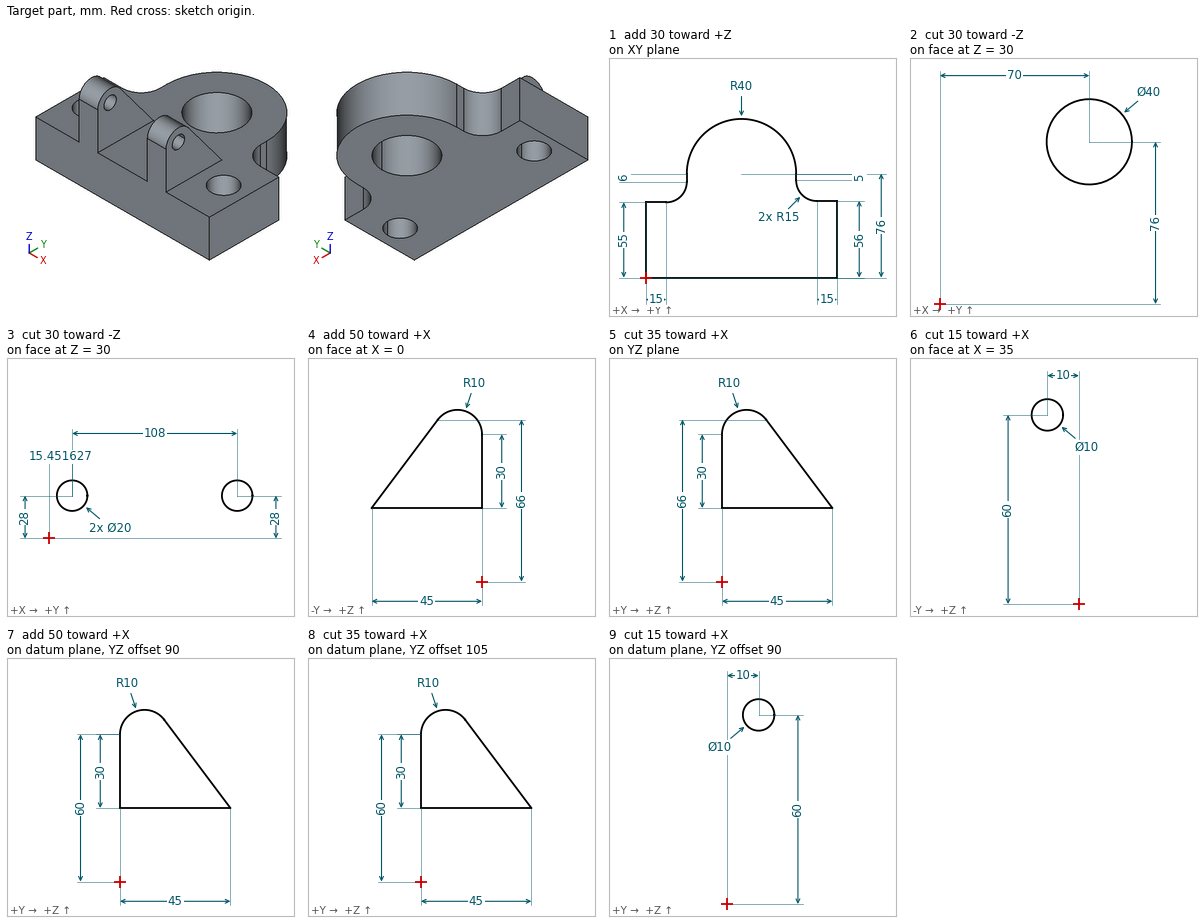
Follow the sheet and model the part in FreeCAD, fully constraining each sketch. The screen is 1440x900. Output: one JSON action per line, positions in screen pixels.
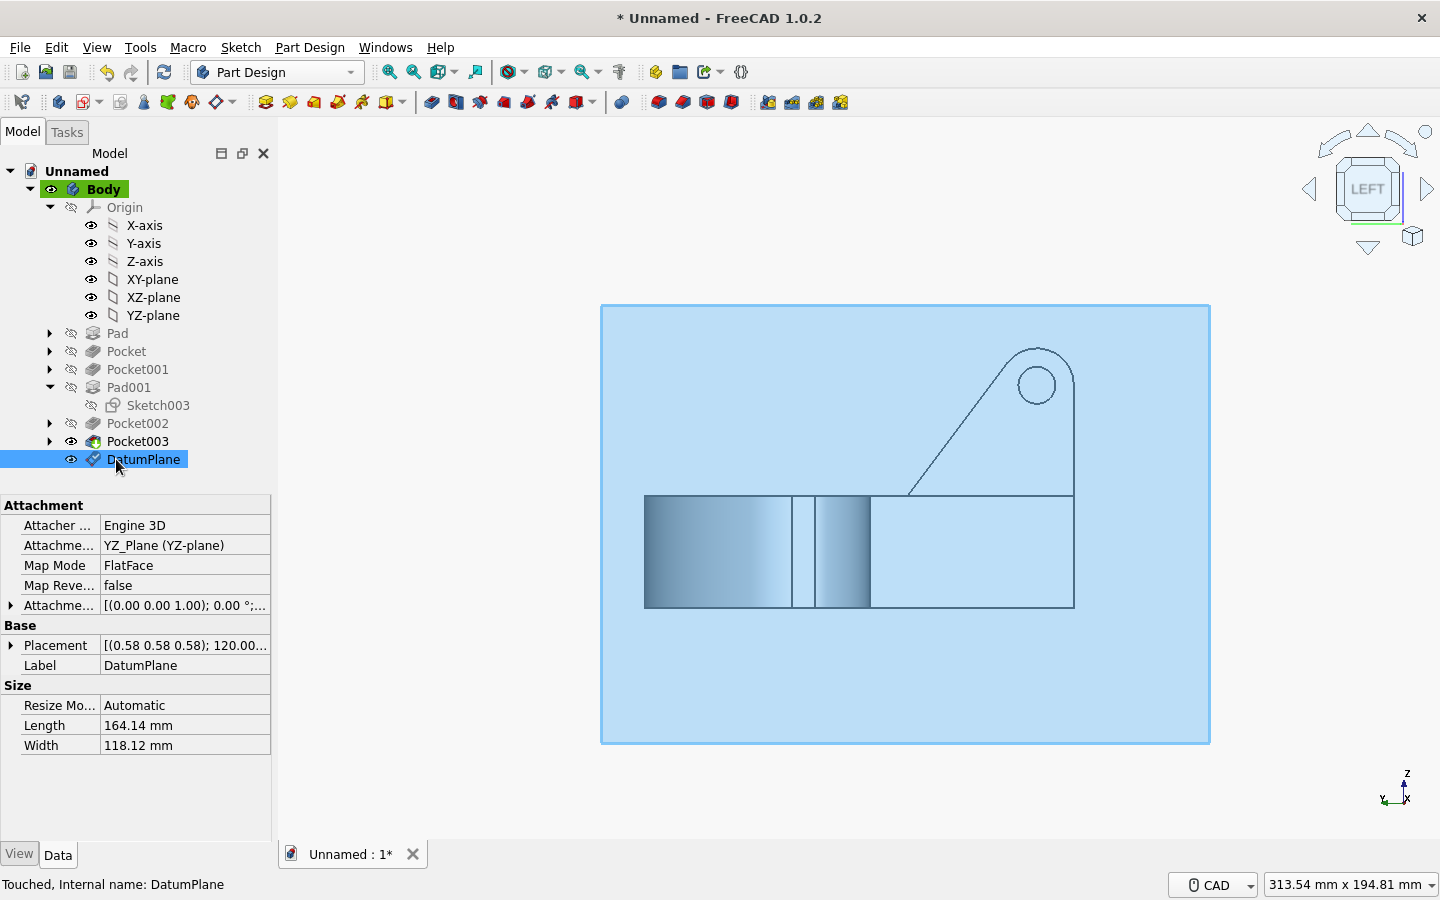
{"action": "left_click", "coordinate": [84, 102]}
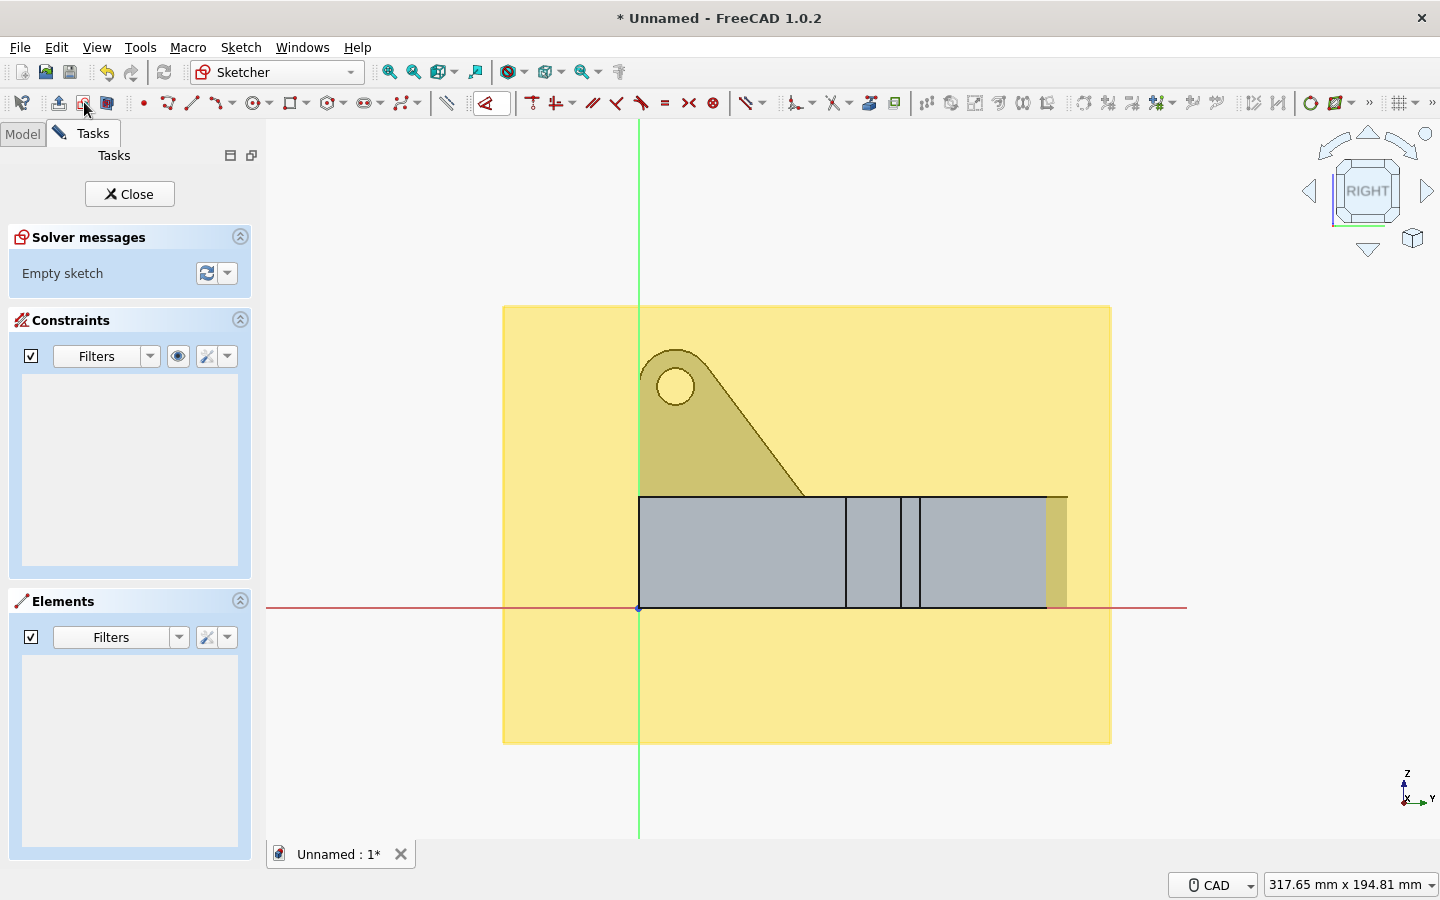
{"action": "left_click", "coordinate": [108, 104]}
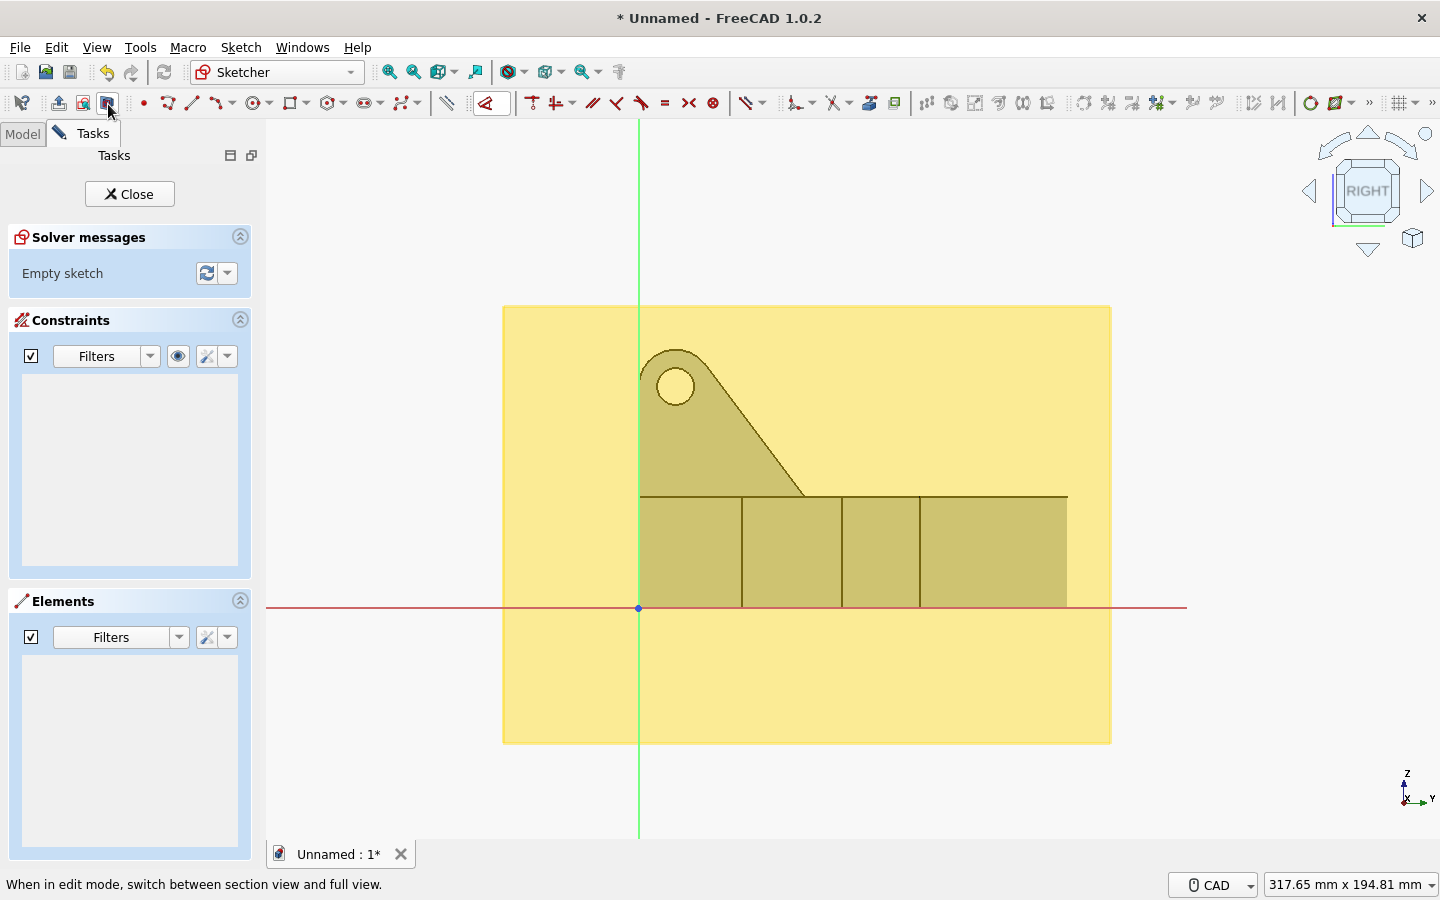
{"action": "scroll", "coordinate": [646, 481], "scroll_direction": "up", "scroll_amount": 3}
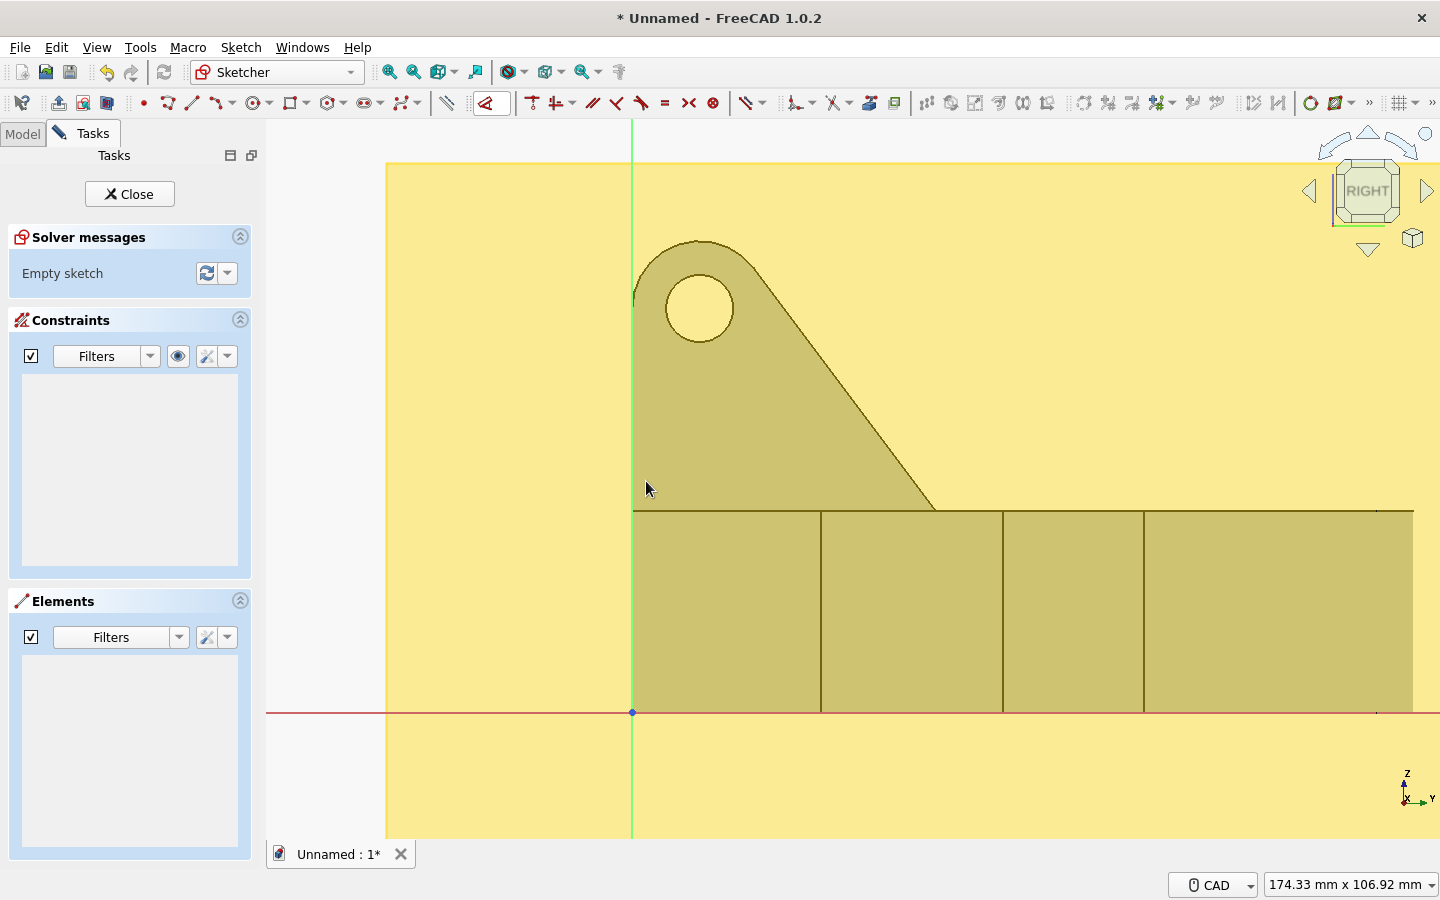
{"action": "key", "text": "g m"}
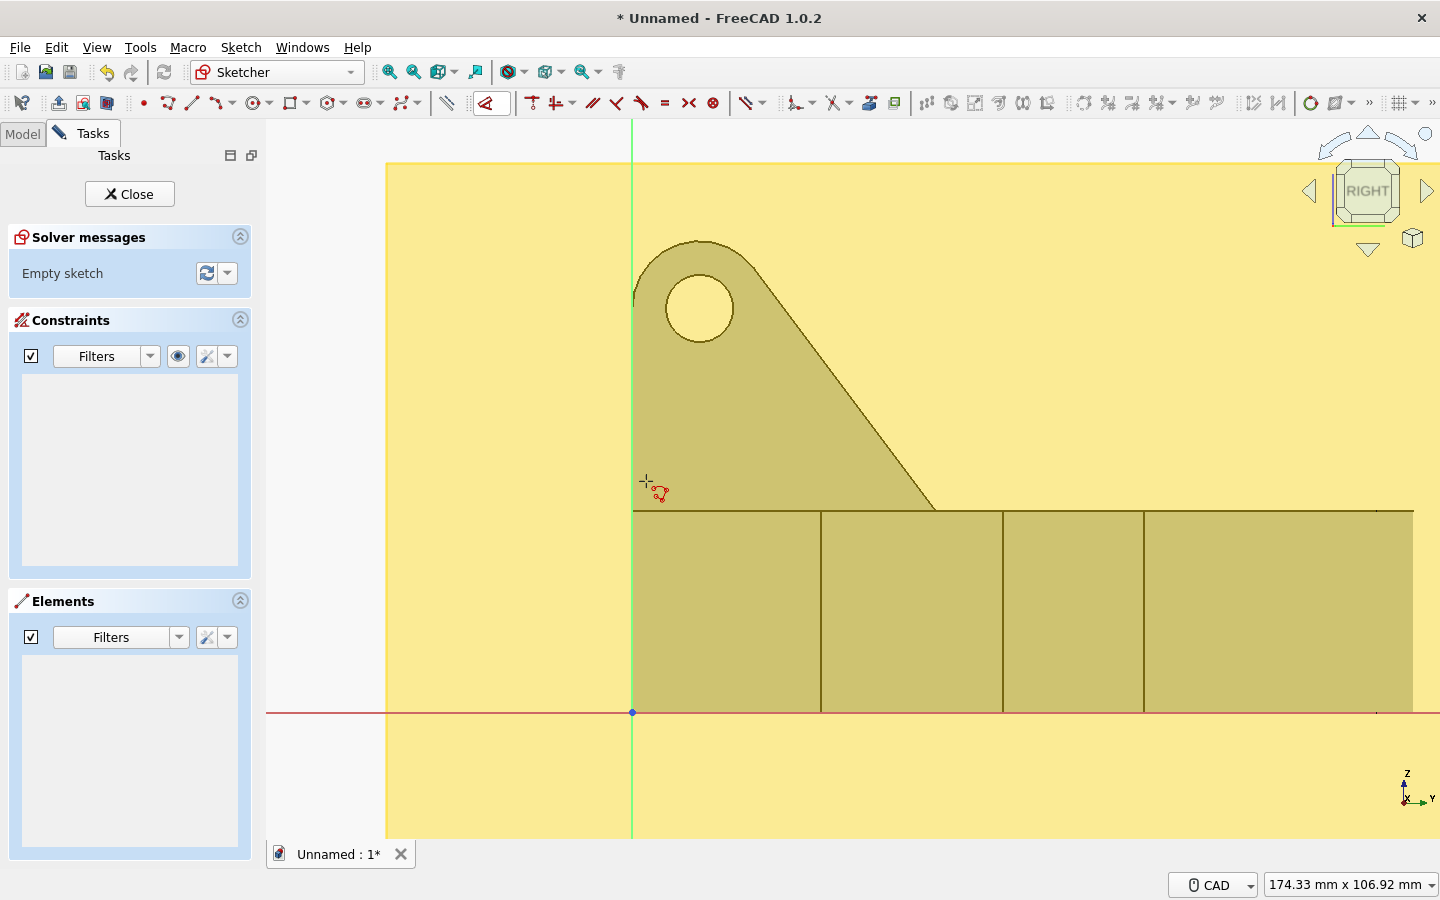
{"action": "left_click", "coordinate": [632, 308]}
{"action": "left_click", "coordinate": [641, 511]}
{"action": "left_click", "coordinate": [935, 511]}
{"action": "left_click", "coordinate": [754, 268]}
{"action": "right_click", "coordinate": [754, 268]}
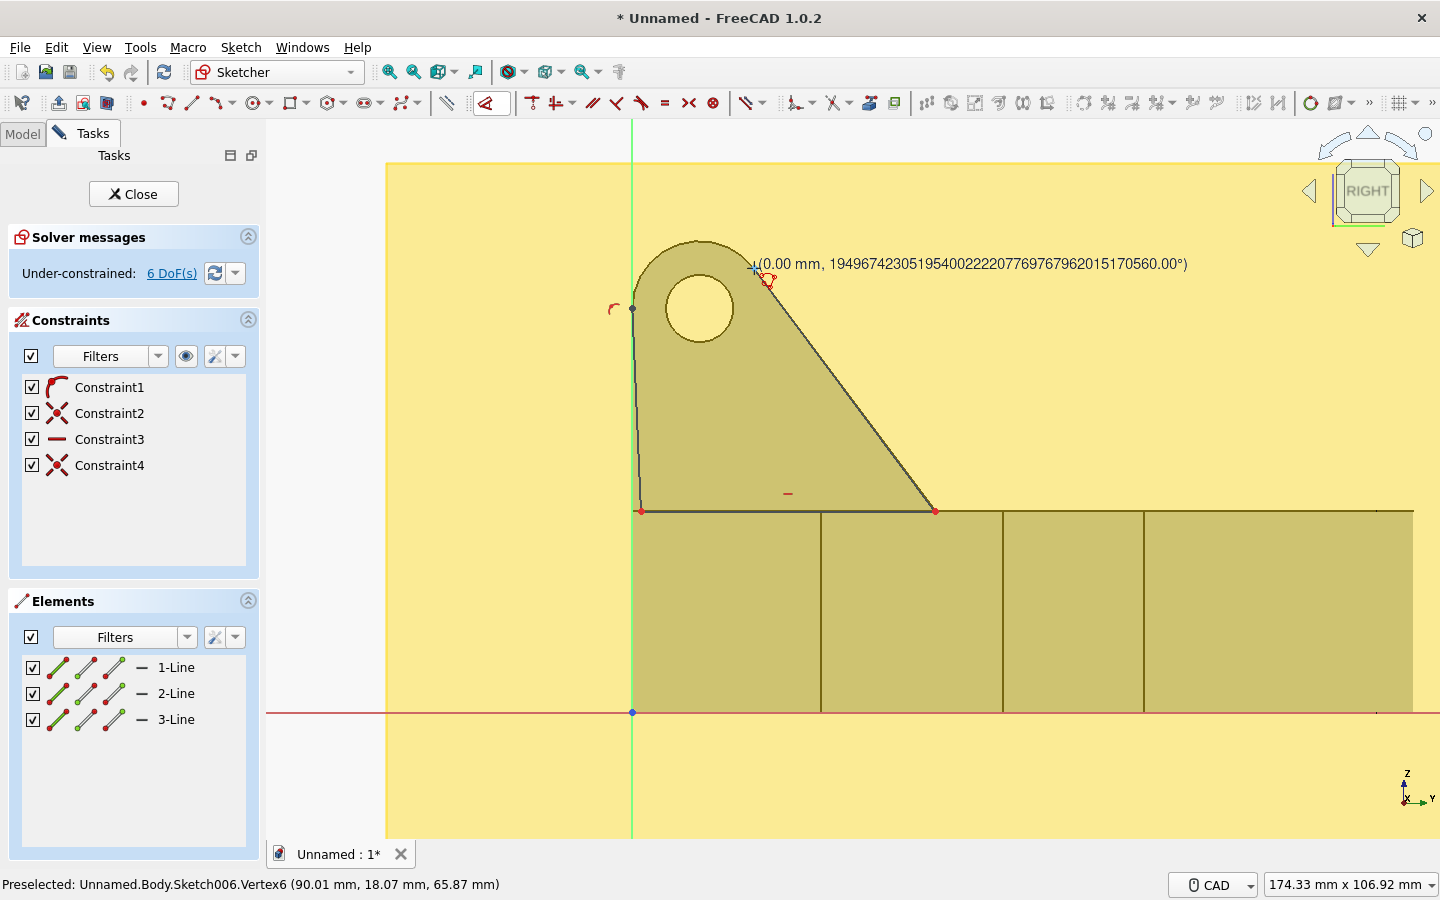
{"action": "key", "text": "g 3 a"}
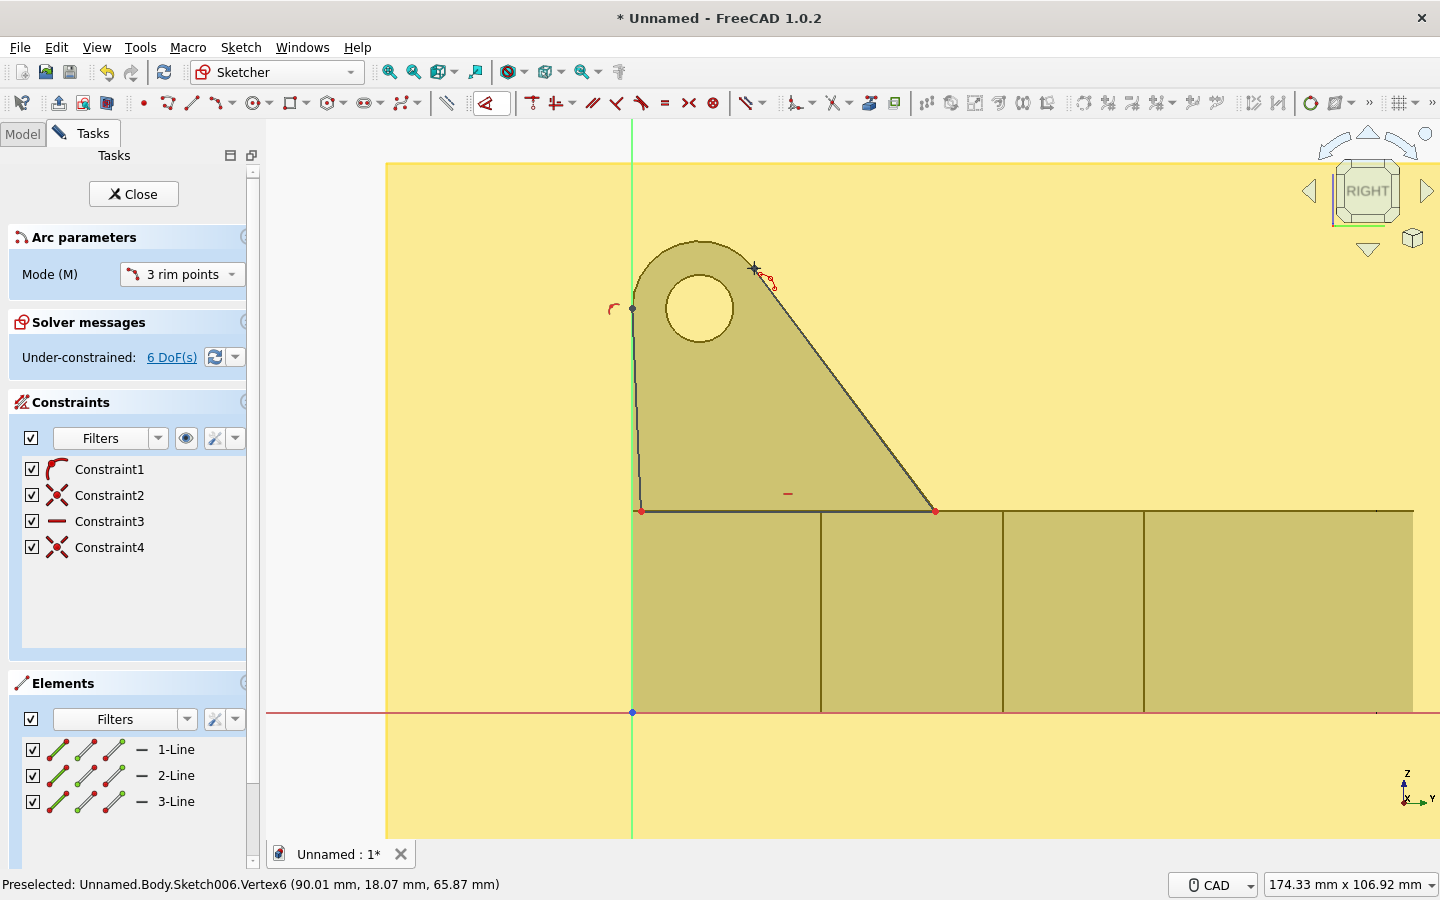
{"action": "left_click", "coordinate": [754, 269]}
{"action": "left_click", "coordinate": [632, 309]}
{"action": "left_click", "coordinate": [678, 245]}
{"action": "key", "text": "Escape"}